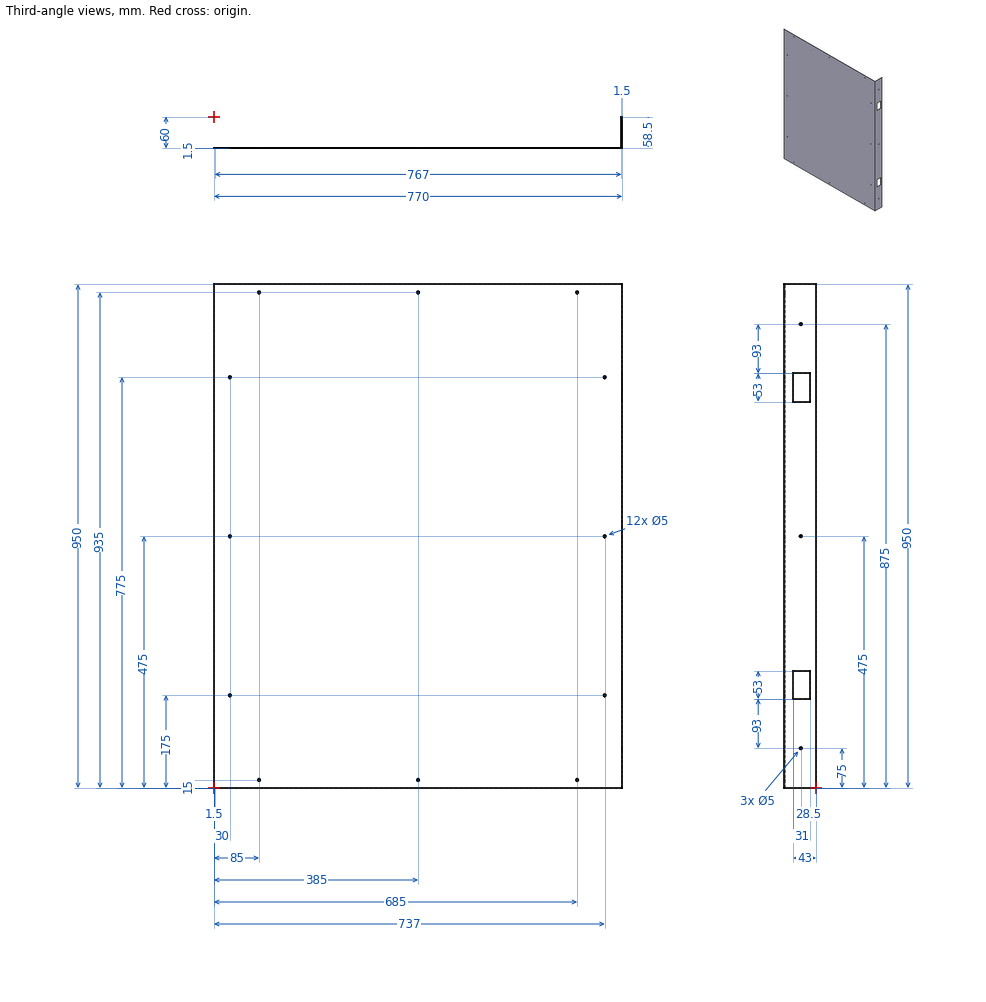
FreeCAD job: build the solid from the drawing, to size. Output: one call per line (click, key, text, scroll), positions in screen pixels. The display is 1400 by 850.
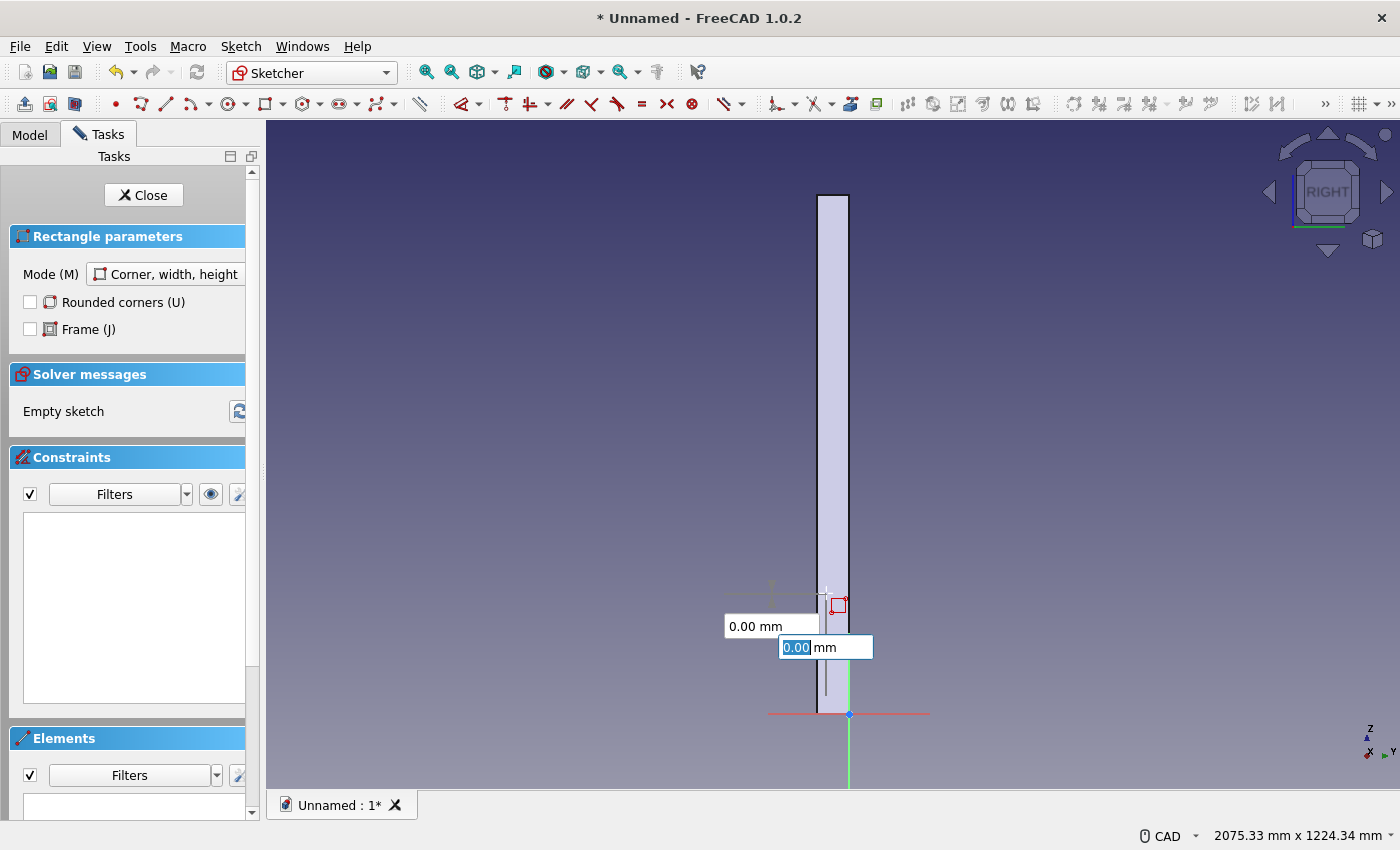
scroll(843, 622, up, 5)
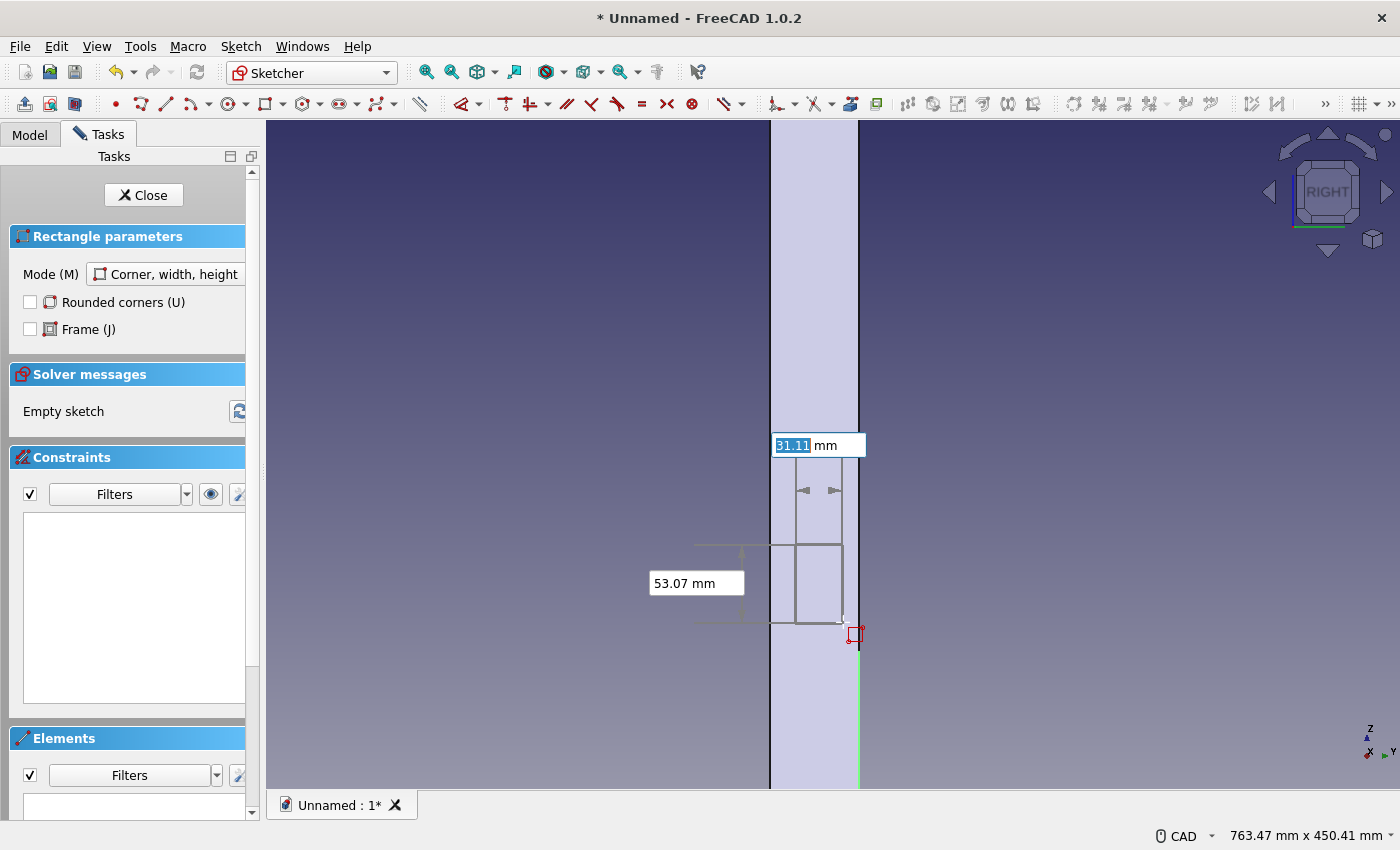
click(842, 621)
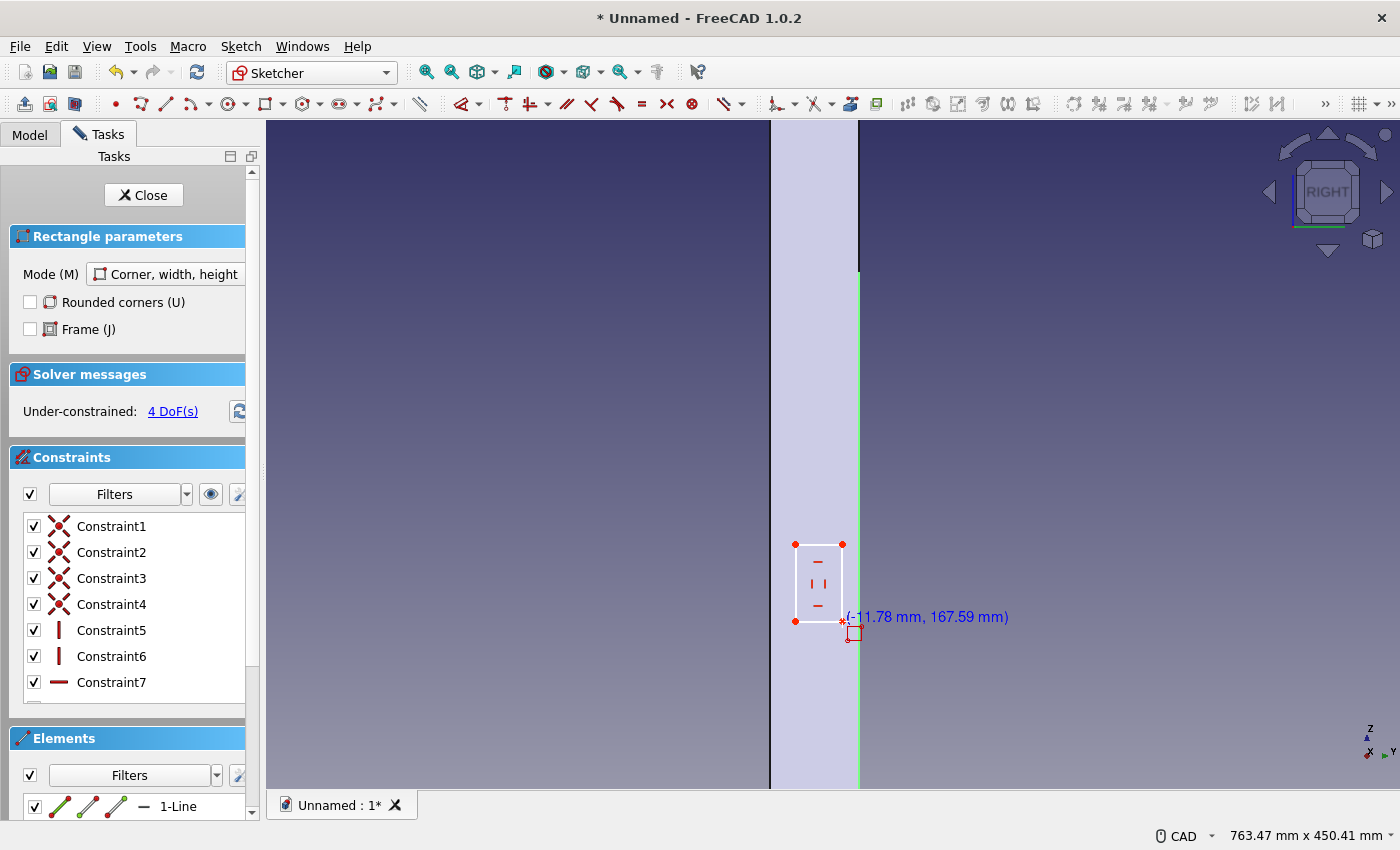
scroll(737, 556, down, 6)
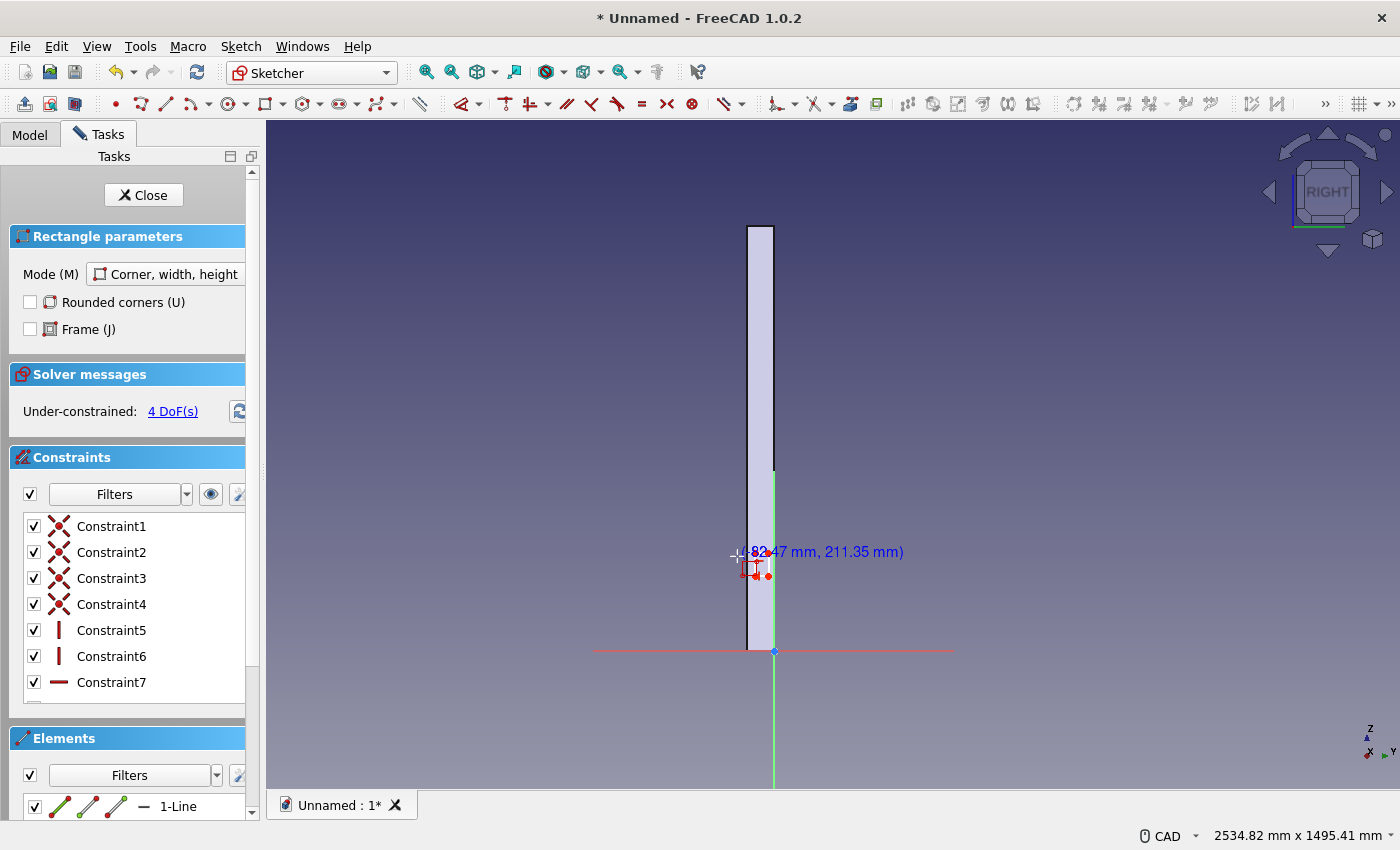
click(755, 301)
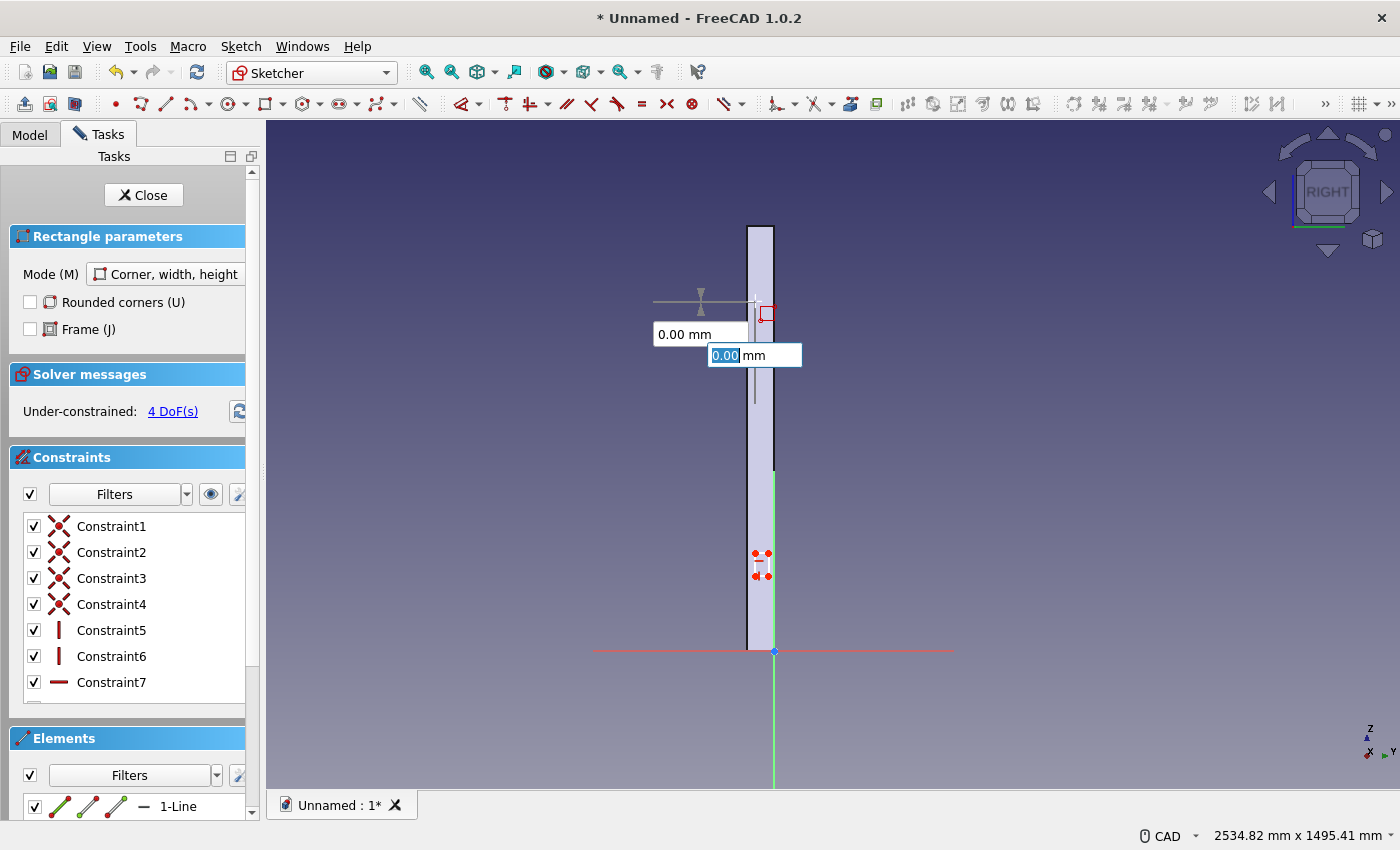
scroll(769, 325, up, 6)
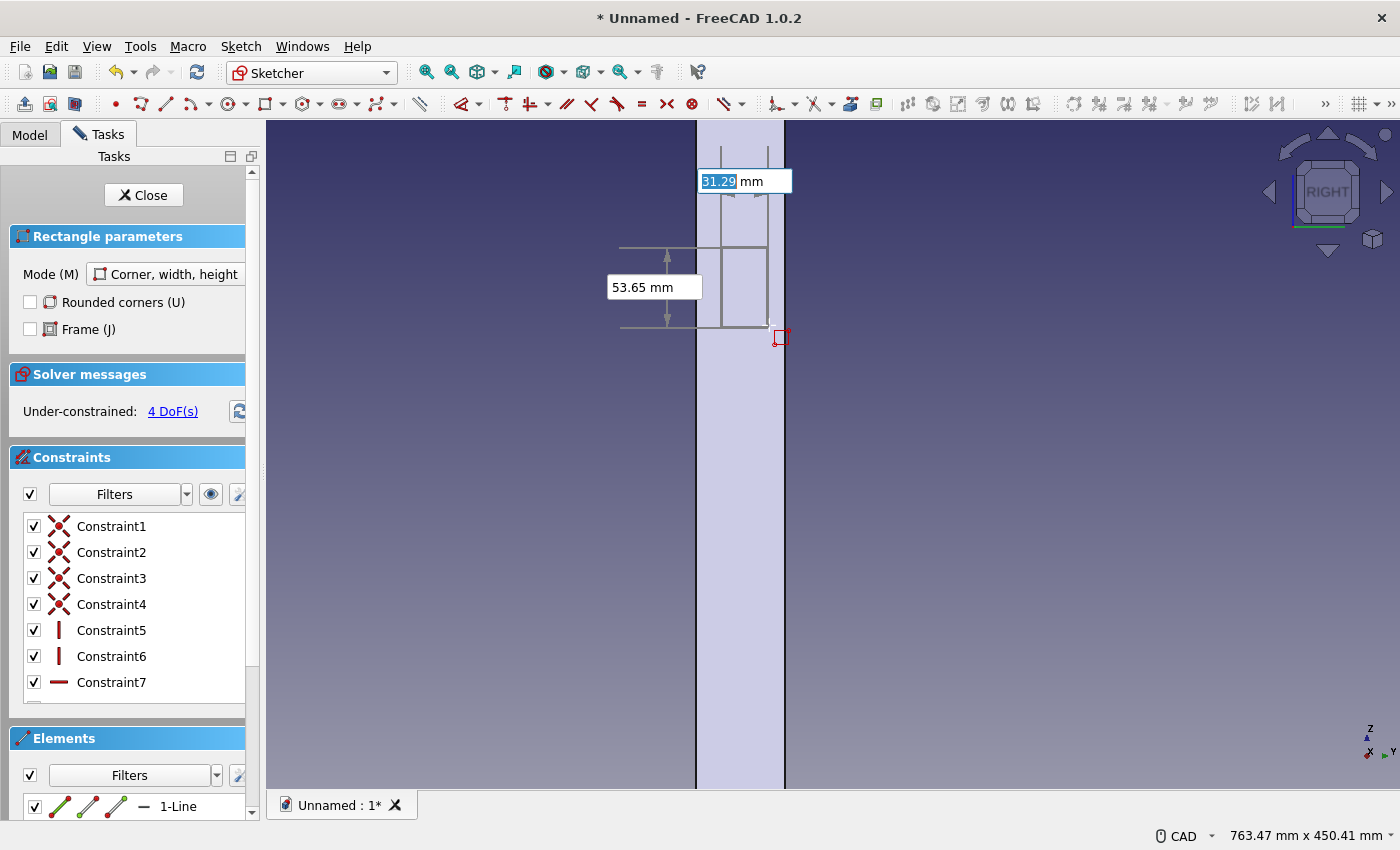
click(767, 325)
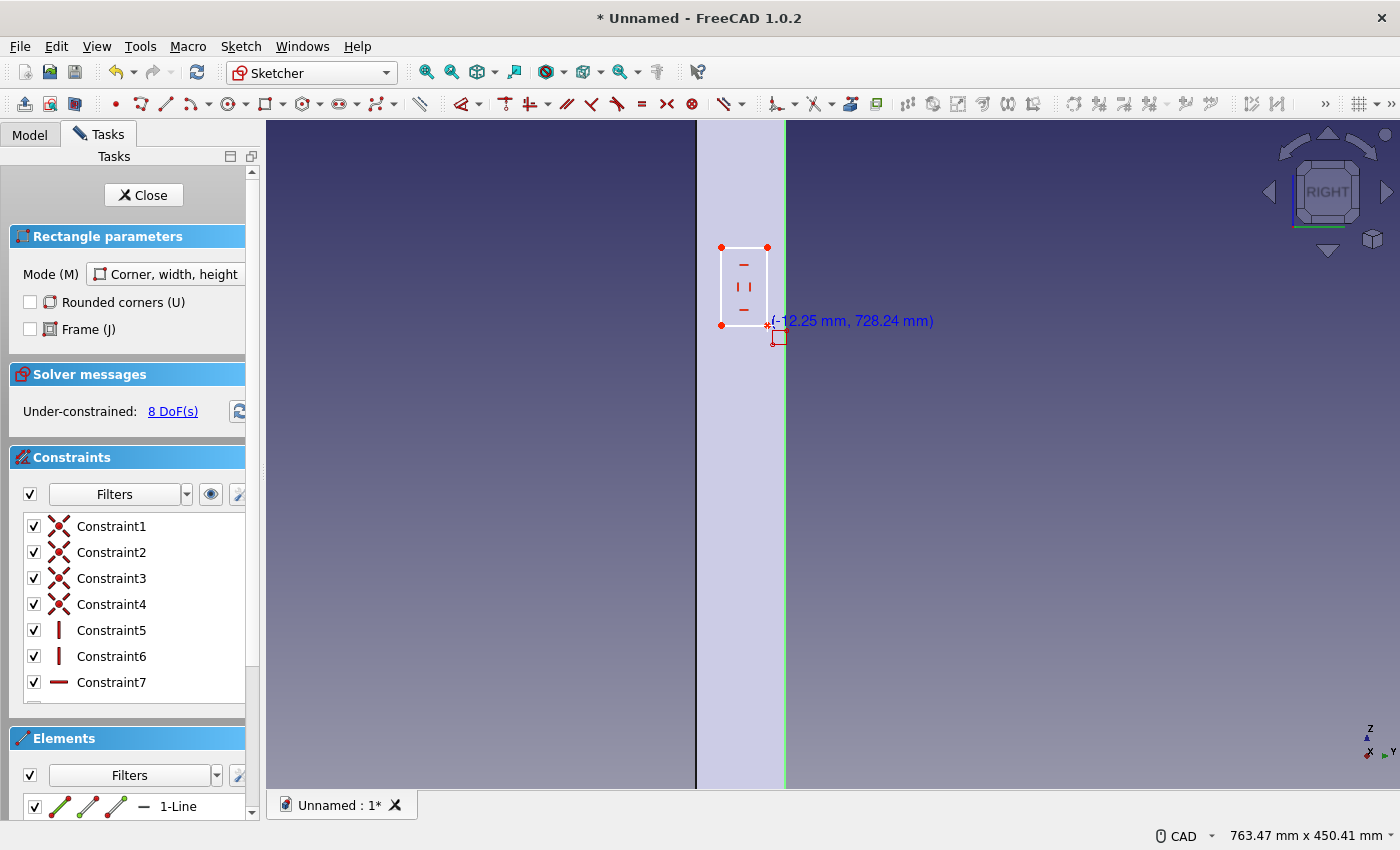
click(228, 104)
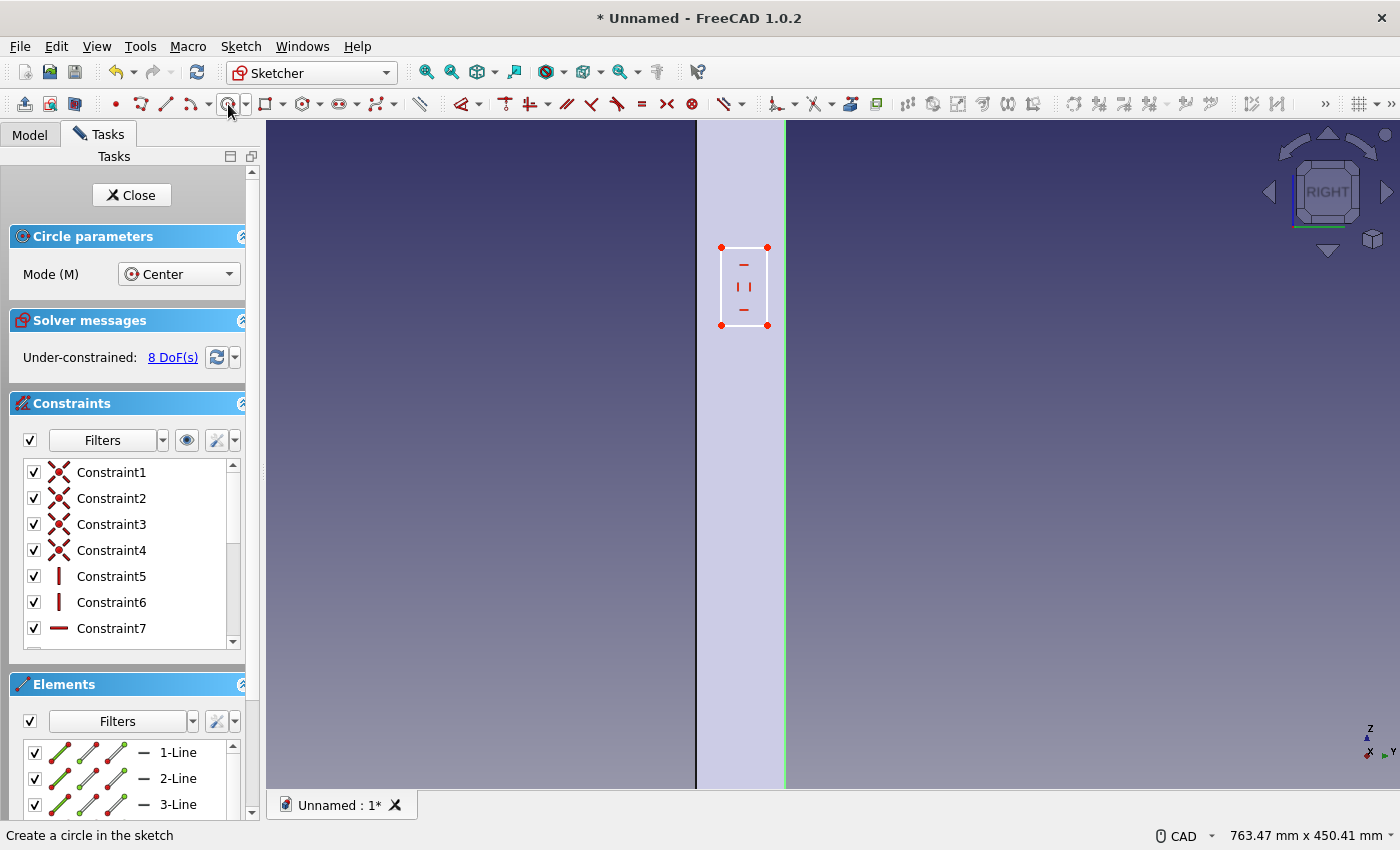
scroll(769, 325, down, 6)